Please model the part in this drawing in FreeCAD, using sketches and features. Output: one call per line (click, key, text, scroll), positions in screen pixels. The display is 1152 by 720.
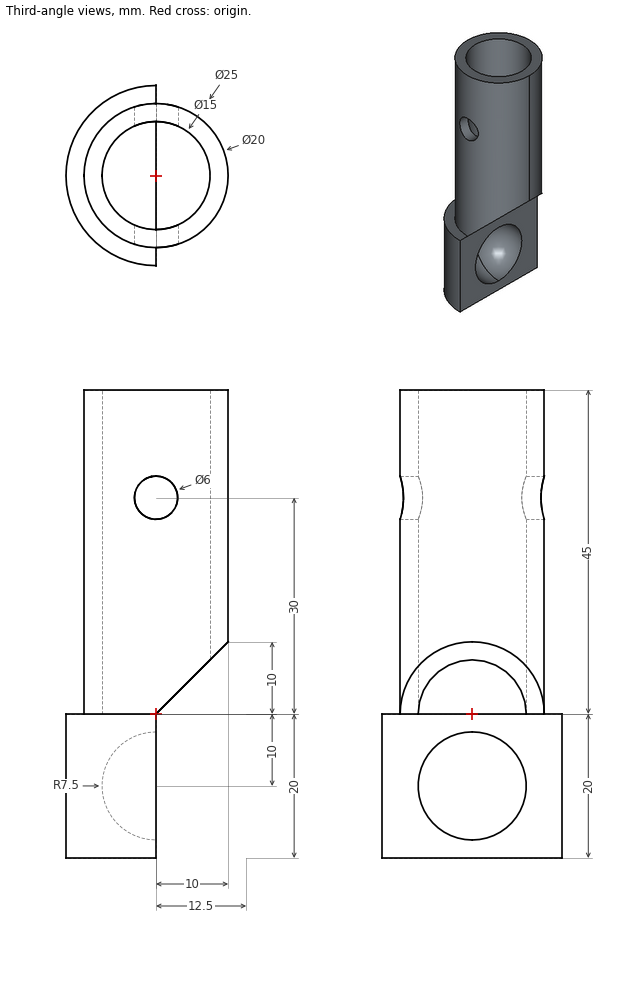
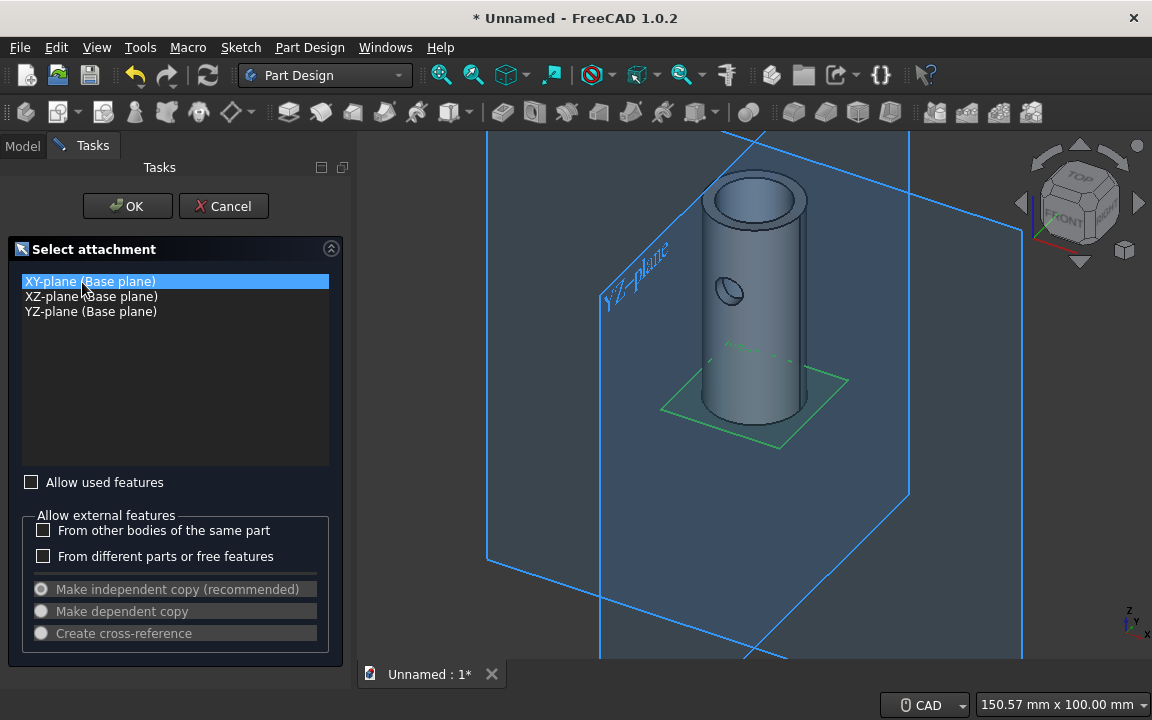
click(128, 206)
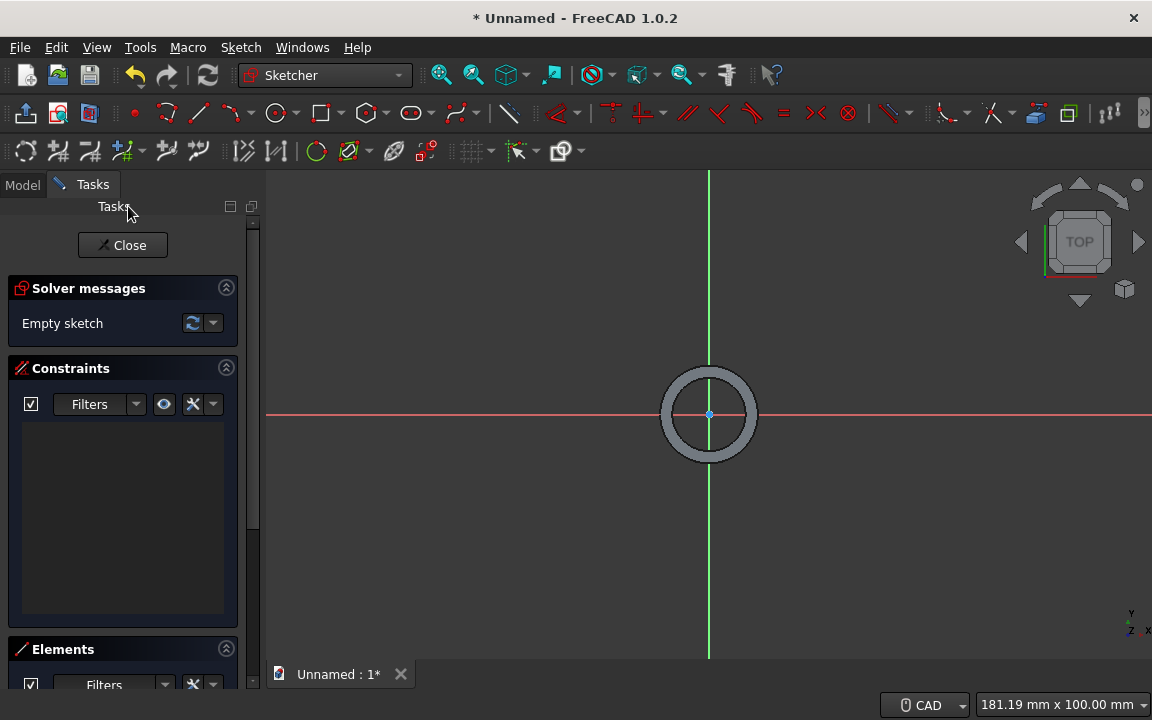
click(90, 114)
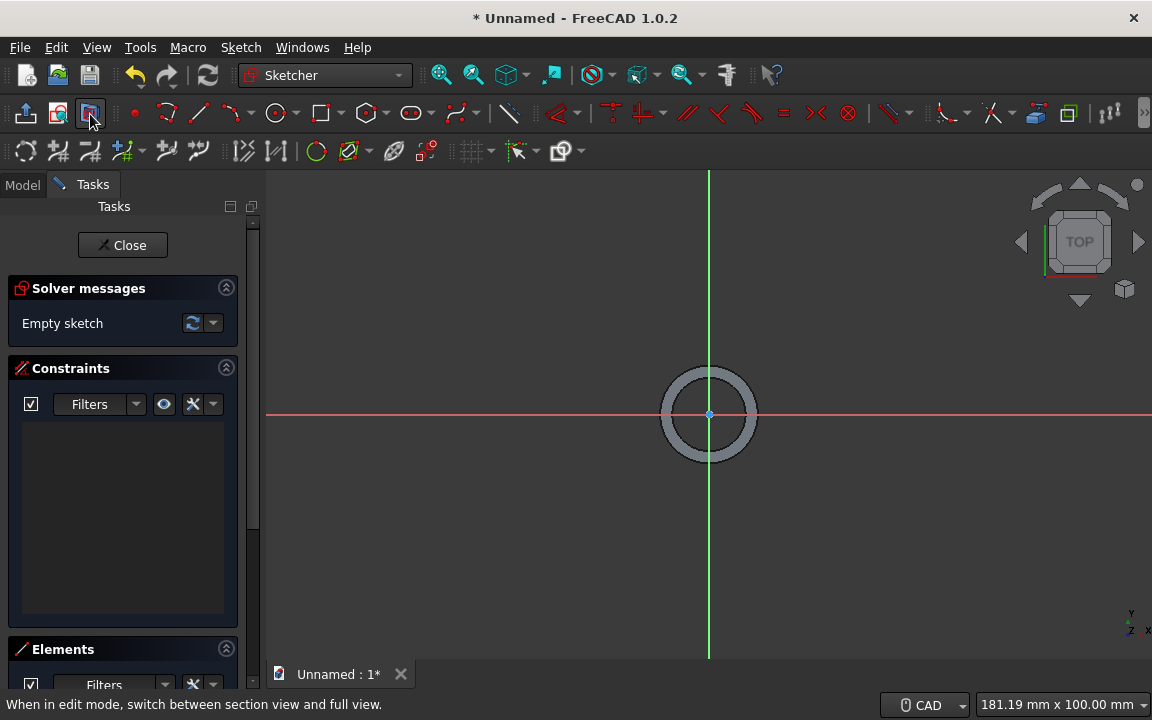
scroll(749, 415, up, 5)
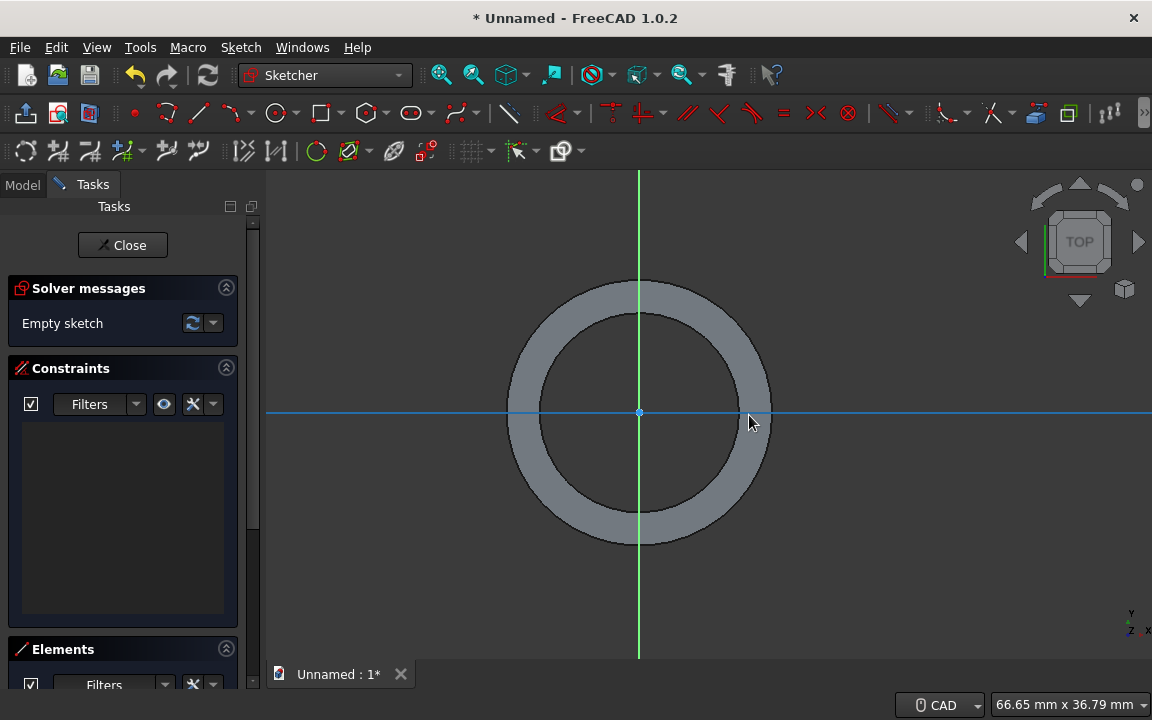
click(276, 114)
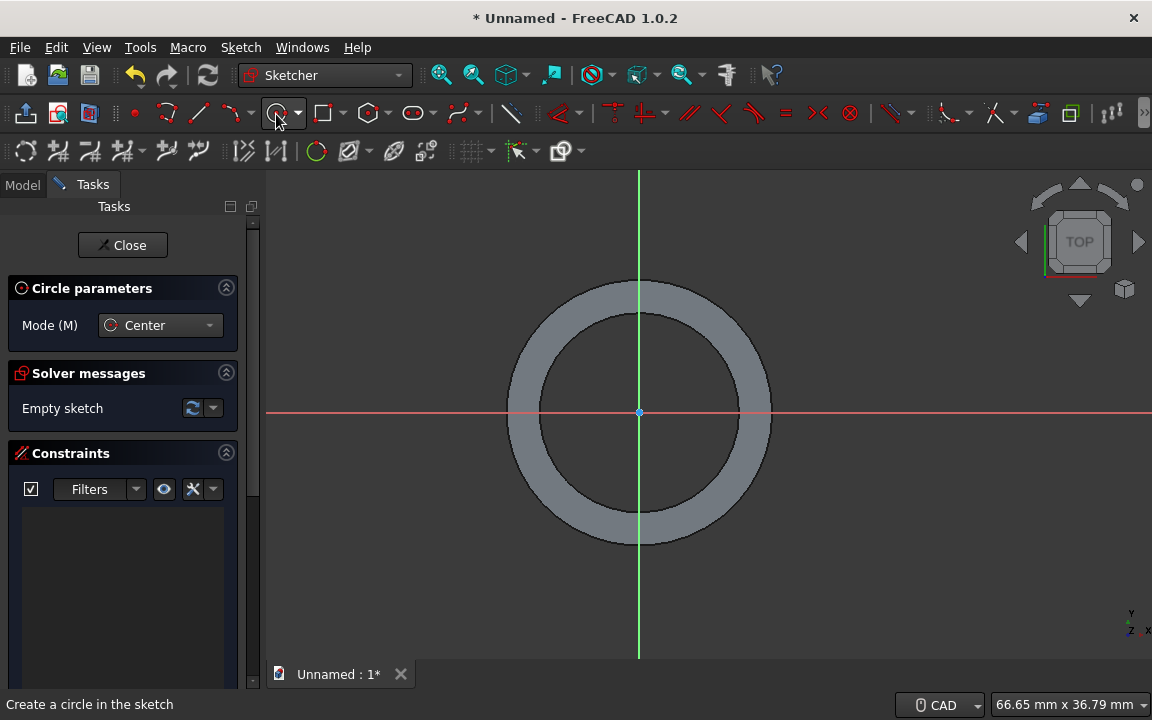
click(639, 413)
click(757, 295)
key(Escape)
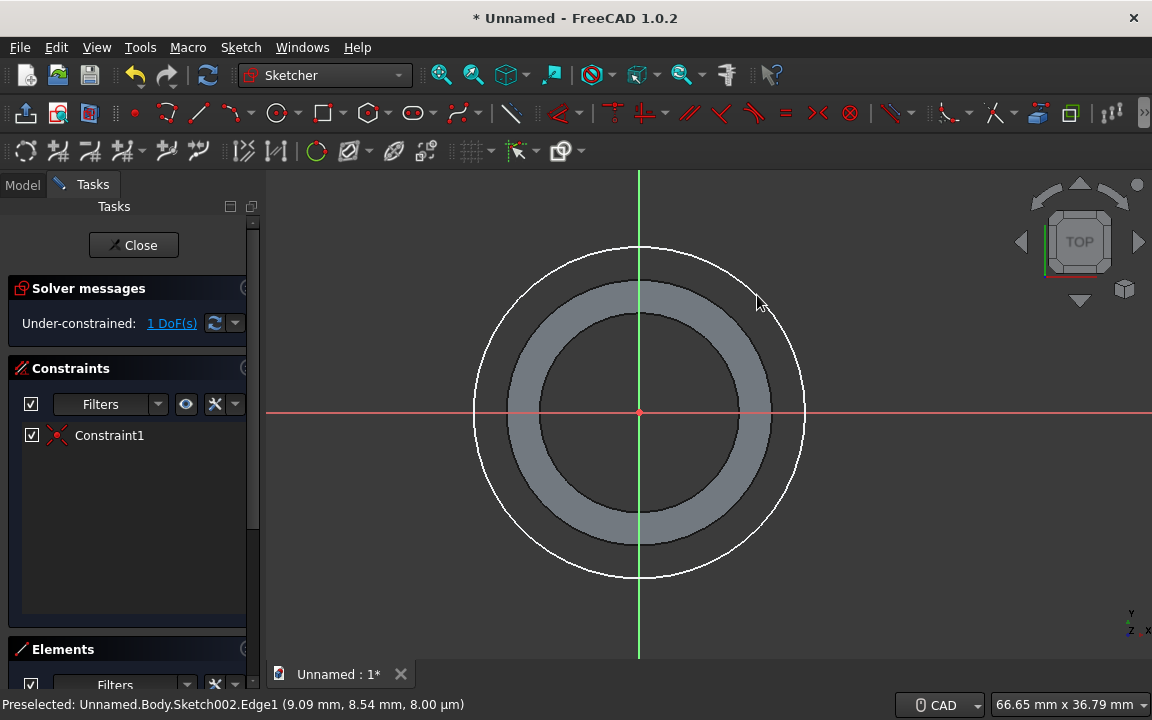
click(558, 114)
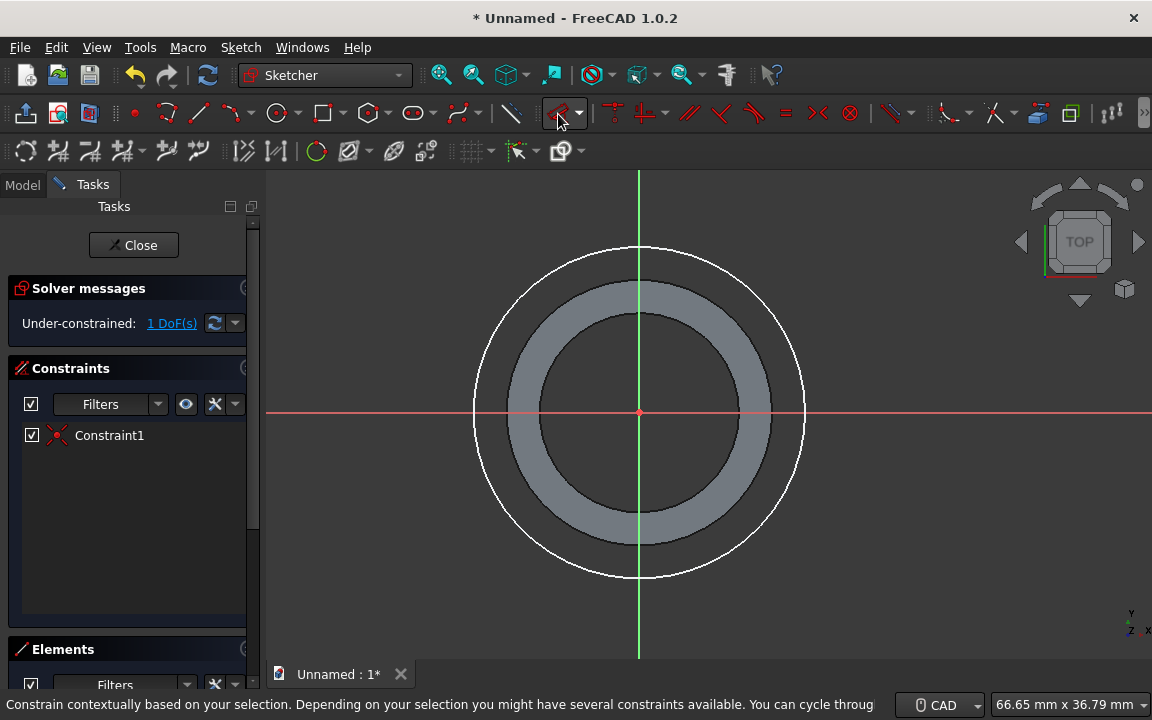
click(756, 295)
click(779, 272)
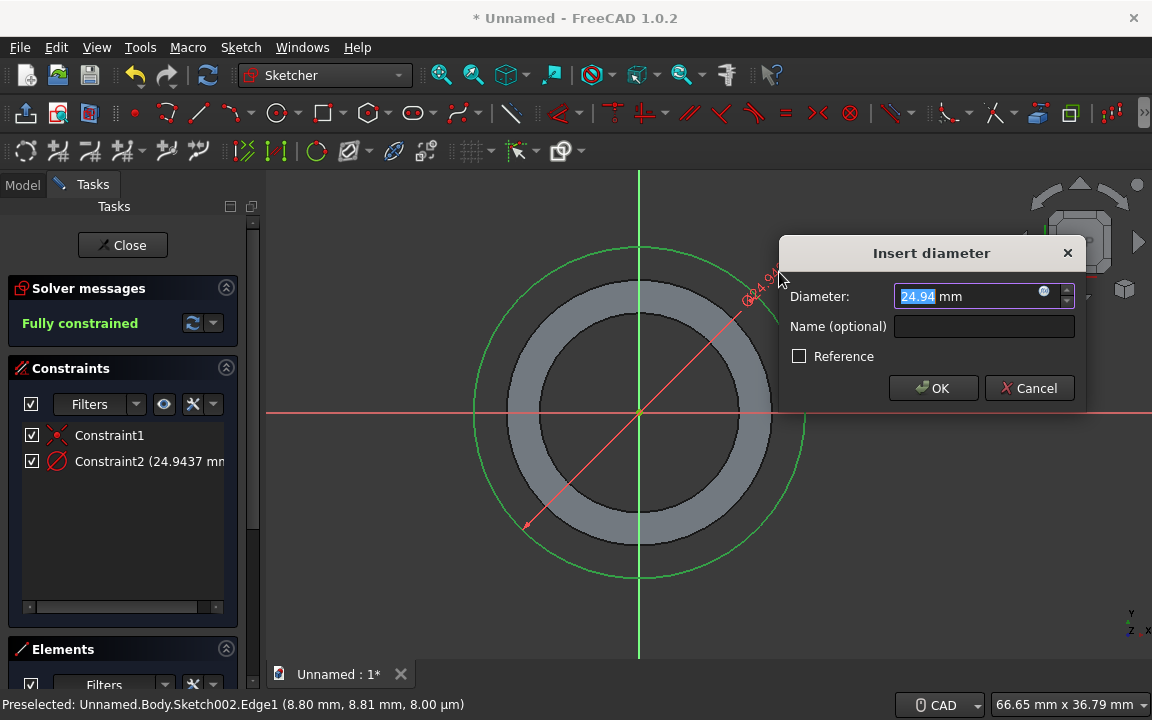
text(25)
key(Return)
key(Escape)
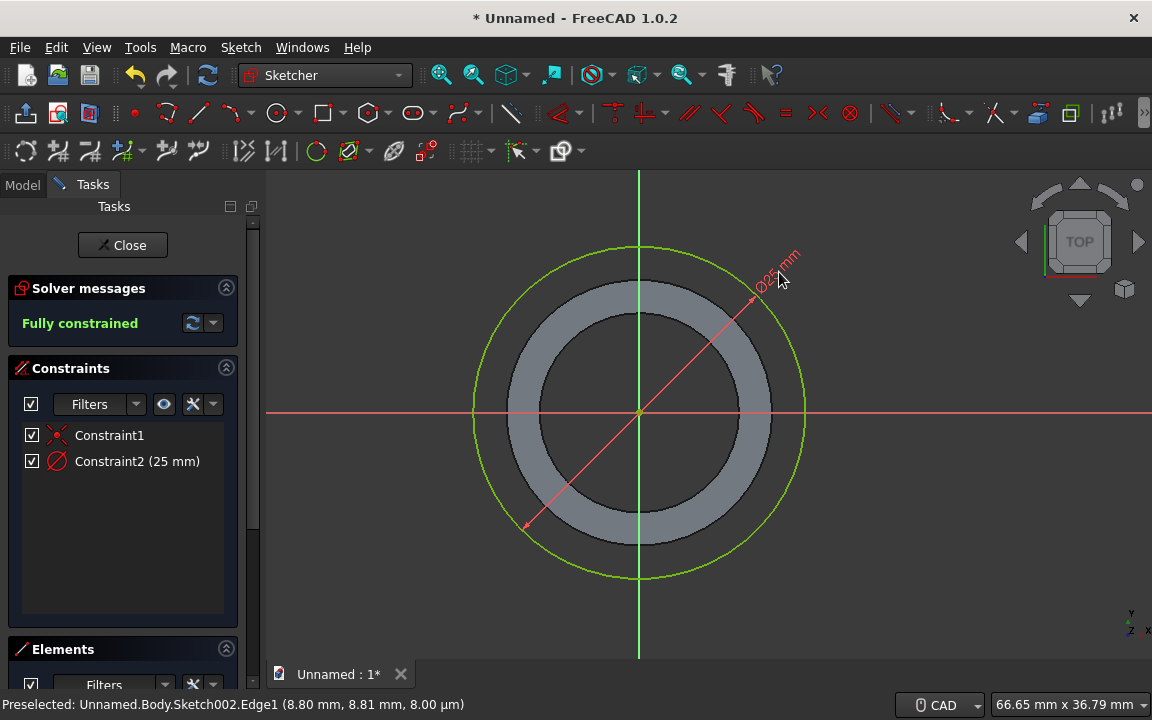
click(123, 245)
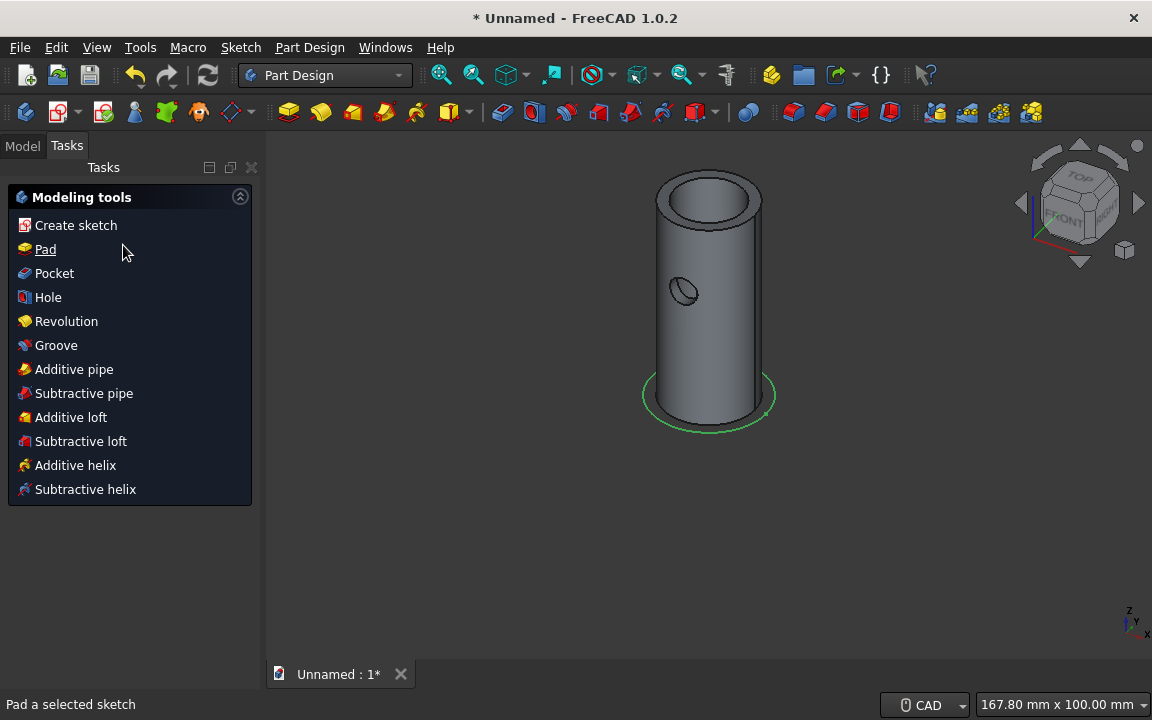
click(290, 112)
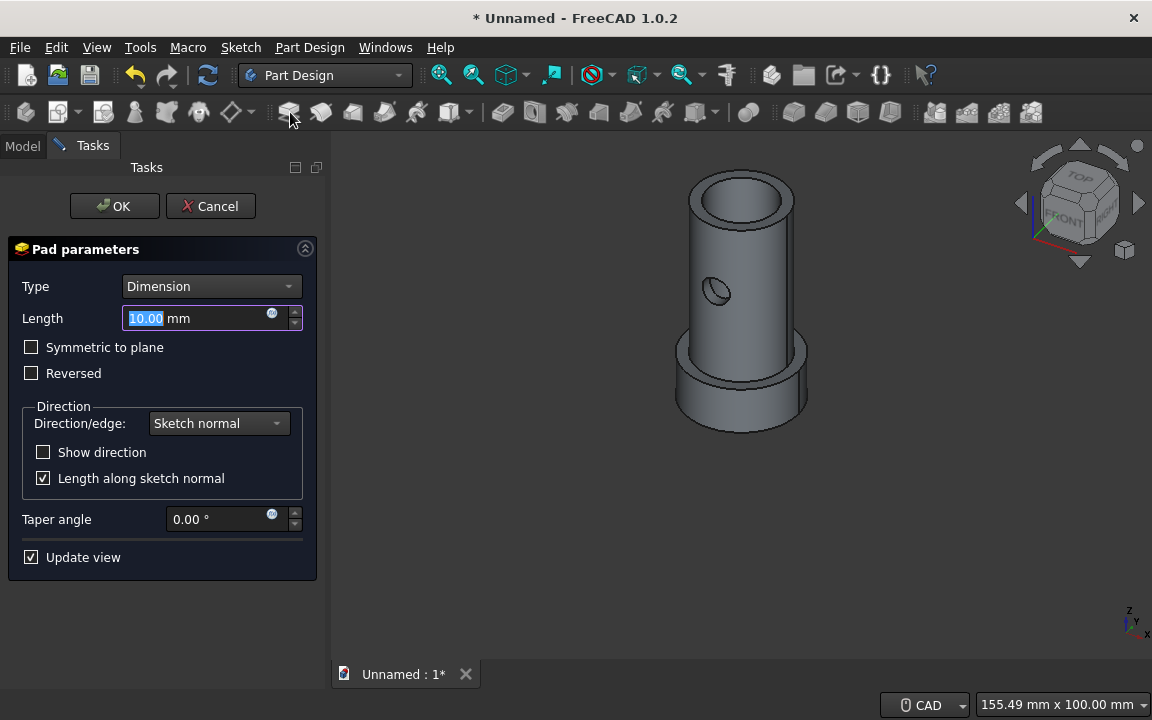
text(20)
key(Tab)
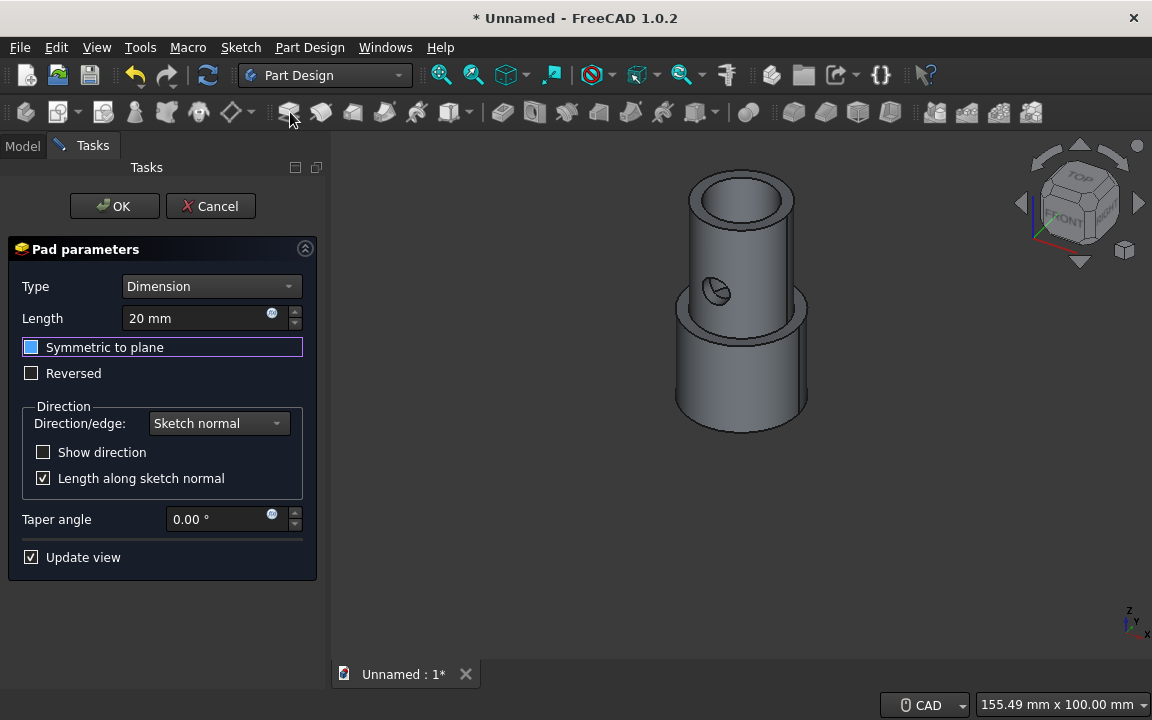
click(30, 373)